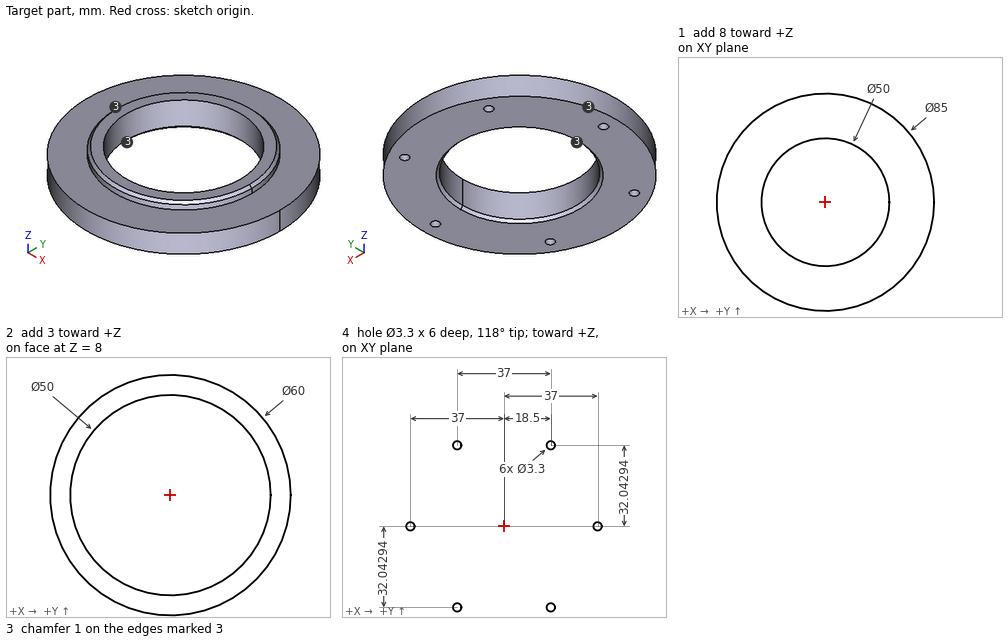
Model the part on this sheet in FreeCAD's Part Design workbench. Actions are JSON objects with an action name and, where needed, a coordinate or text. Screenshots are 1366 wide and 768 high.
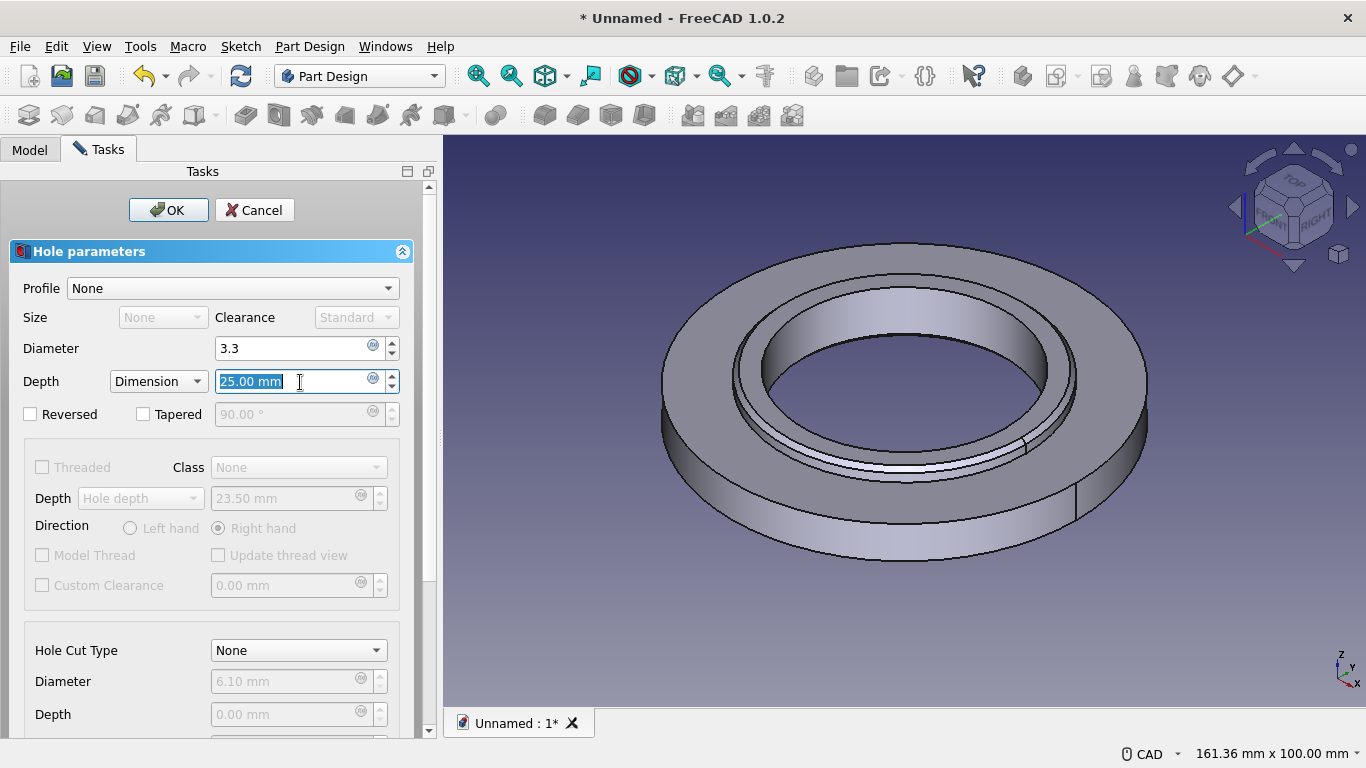
{"action": "type", "text": "6"}
{"action": "key", "text": "Tab"}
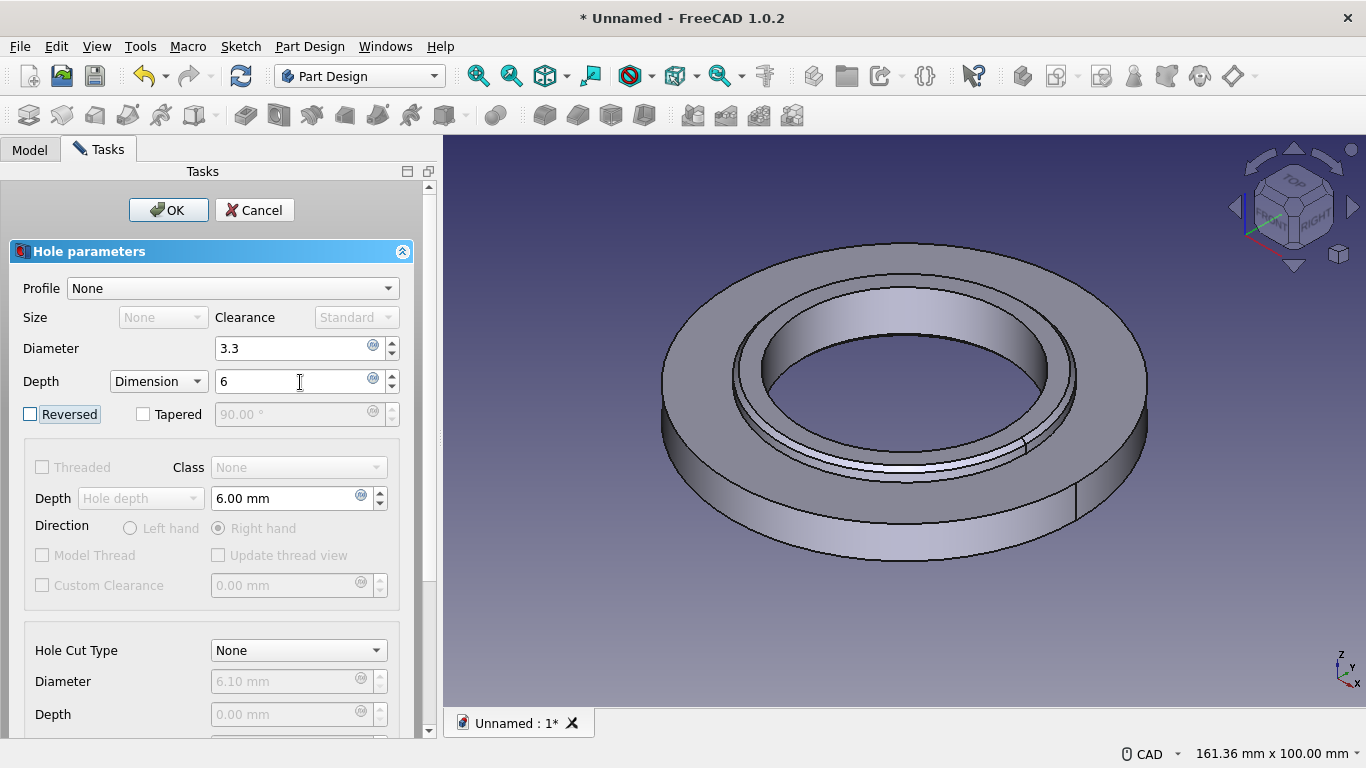
{"action": "left_click", "coordinate": [31, 414]}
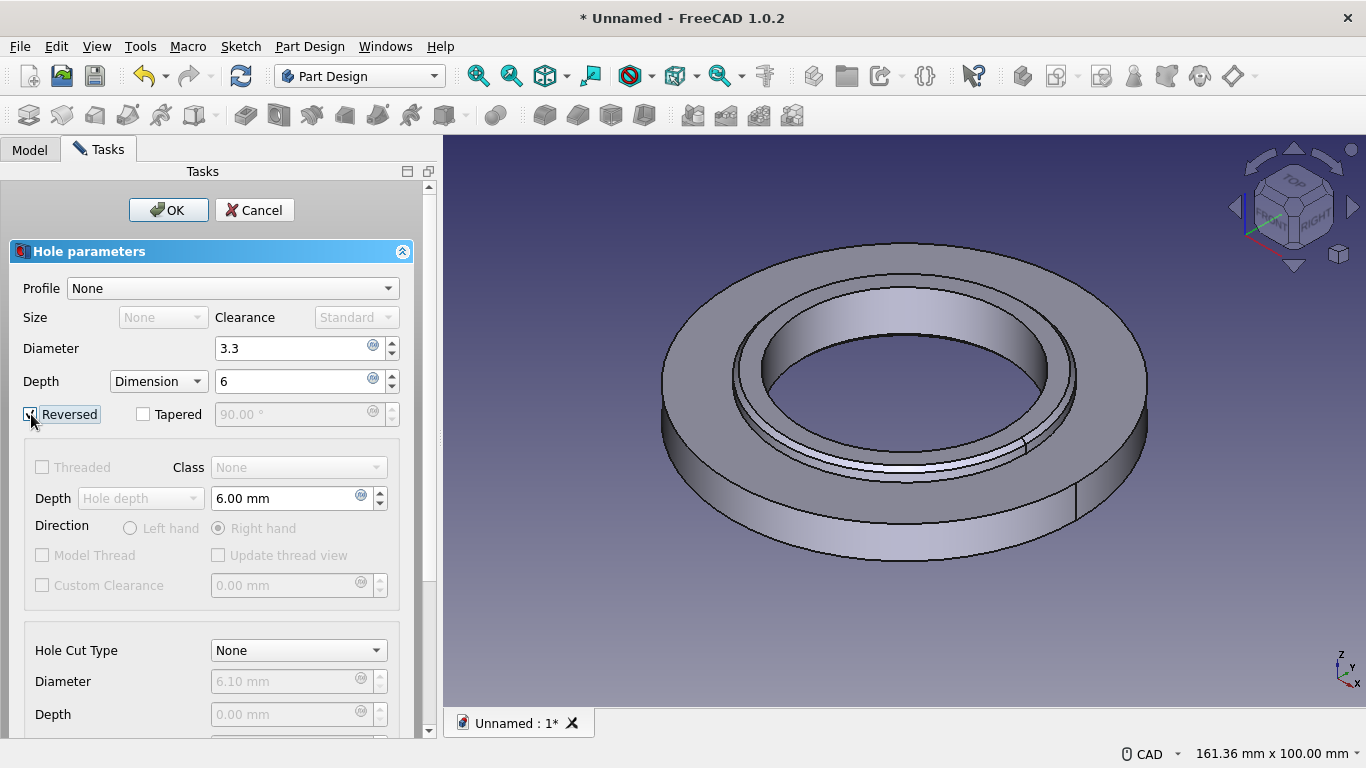
{"action": "left_click", "coordinate": [169, 210]}